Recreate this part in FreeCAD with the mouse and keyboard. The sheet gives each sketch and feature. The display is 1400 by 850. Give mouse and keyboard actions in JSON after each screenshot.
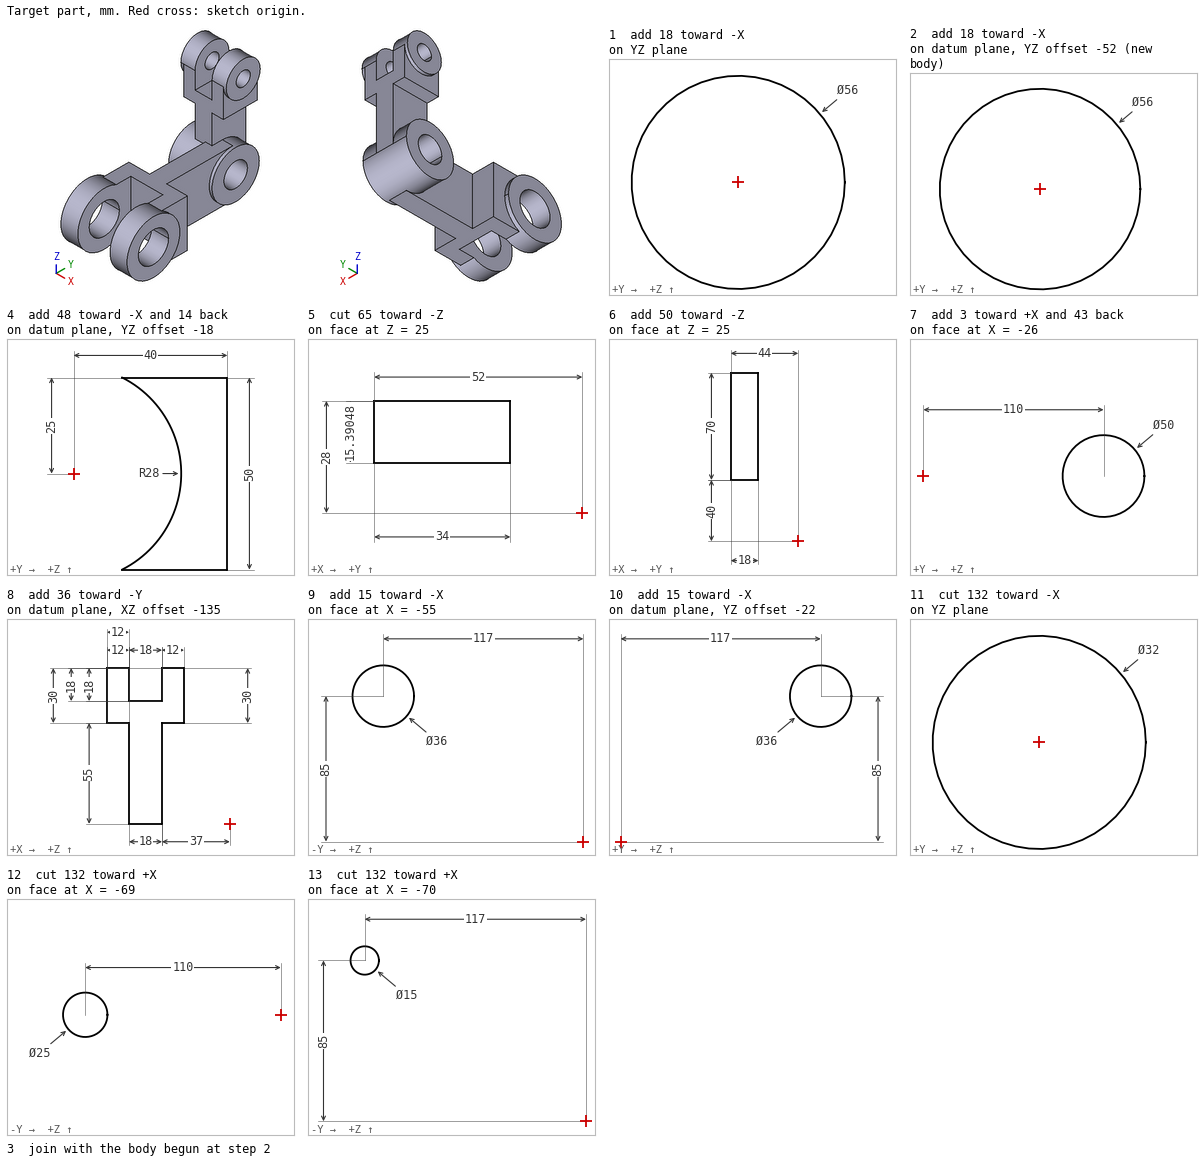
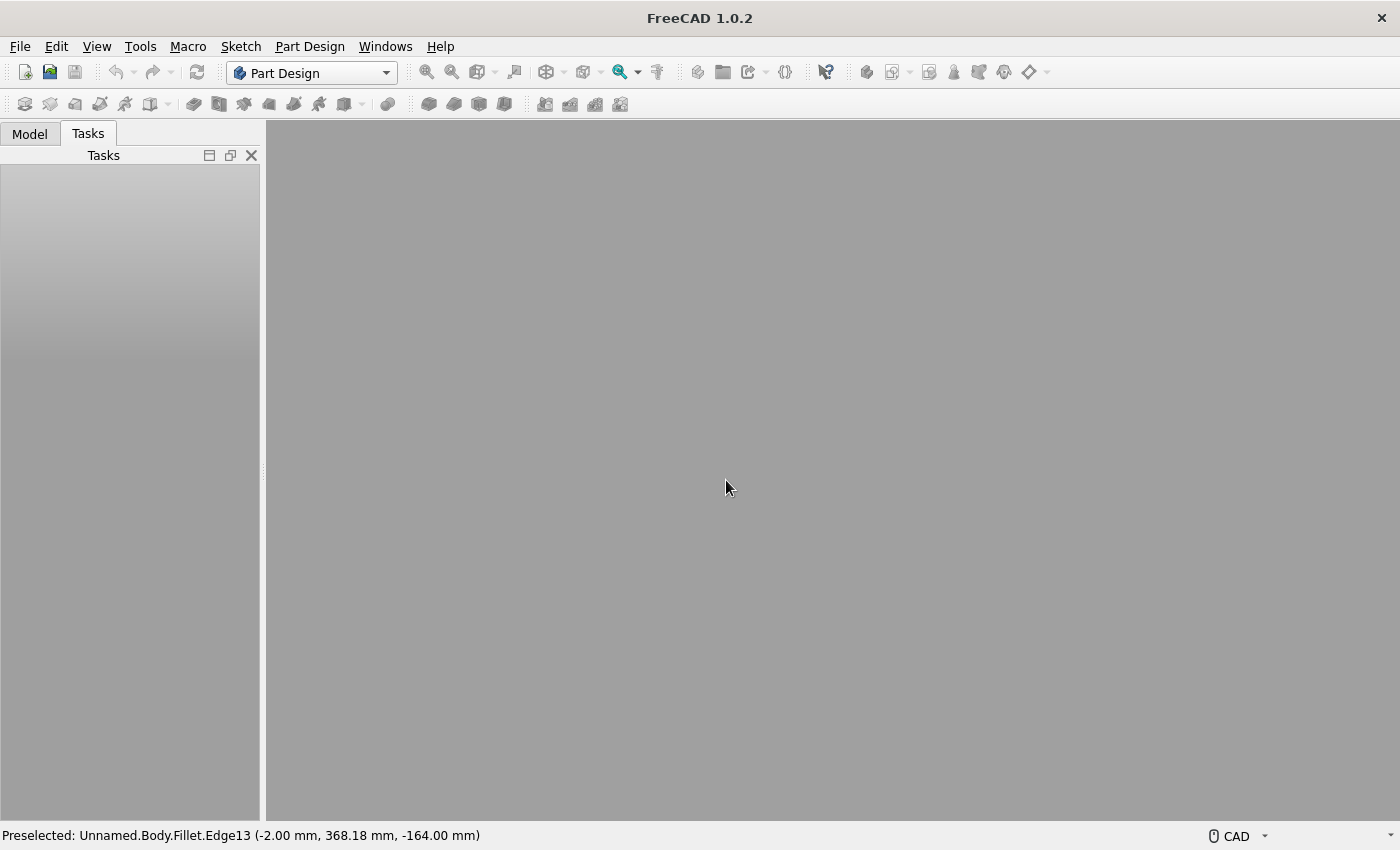
{"action": "key", "text": "ctrl+n"}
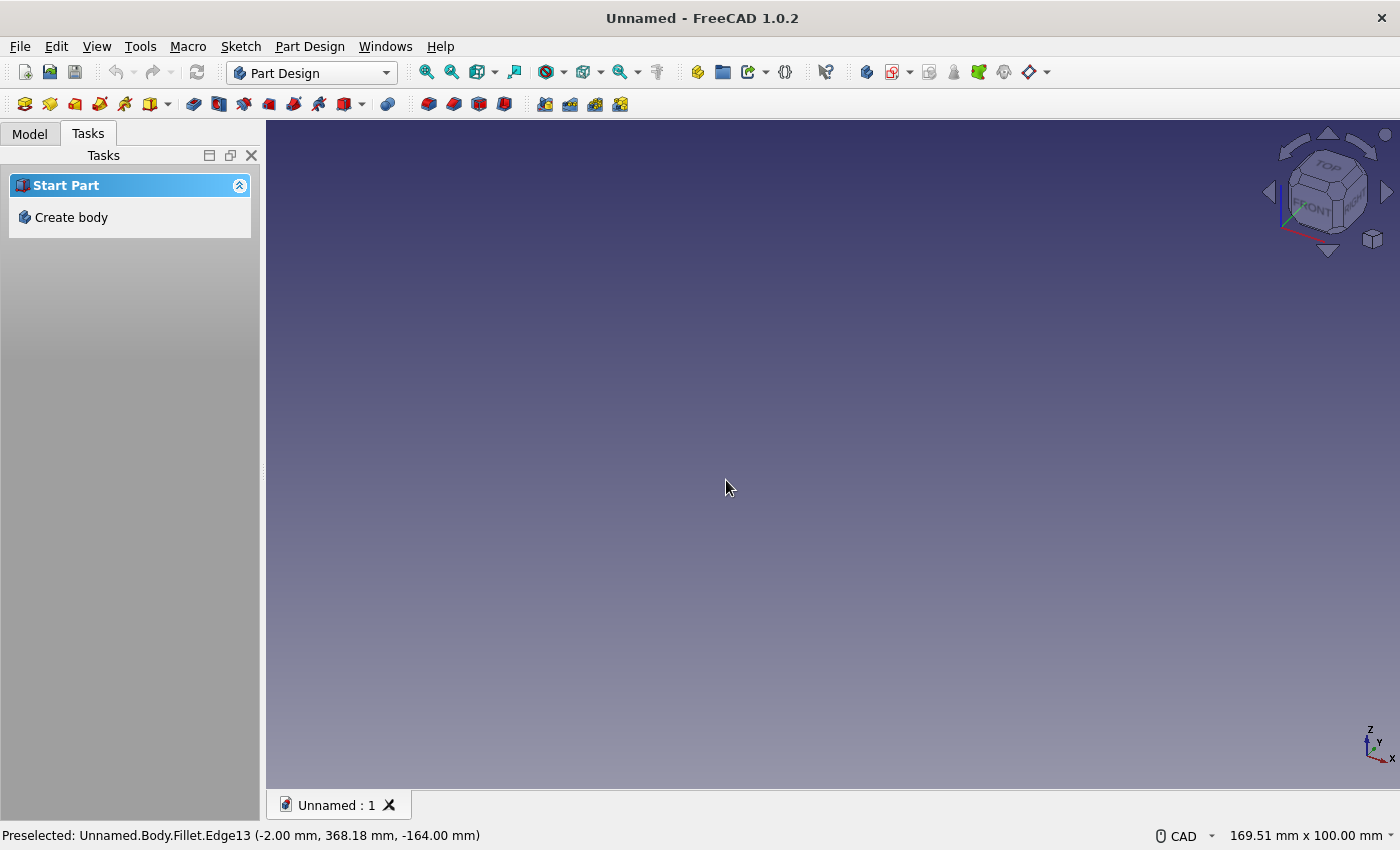
{"action": "left_click", "coordinate": [892, 72]}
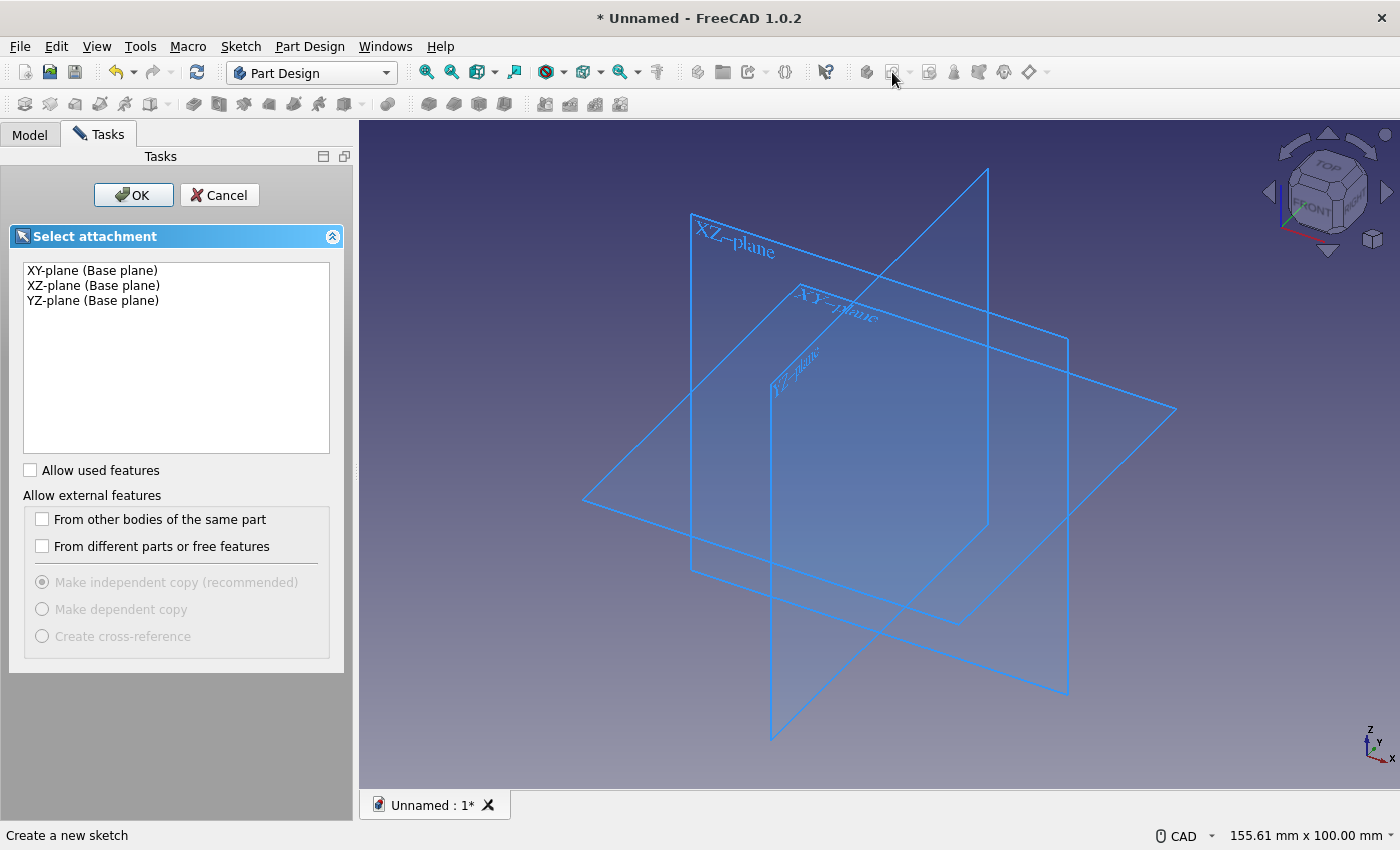
{"action": "left_click", "coordinate": [84, 300]}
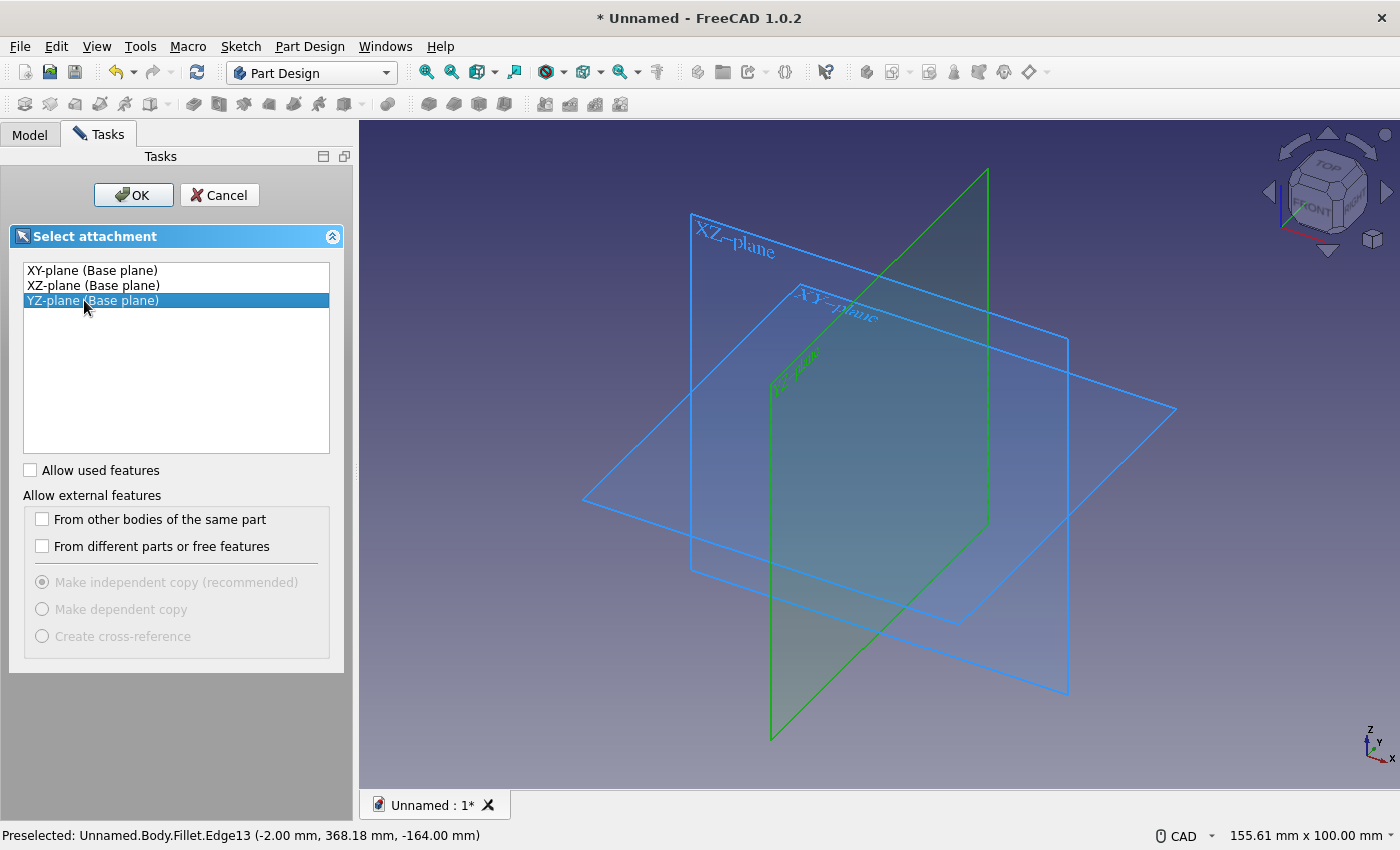
{"action": "left_click", "coordinate": [134, 195]}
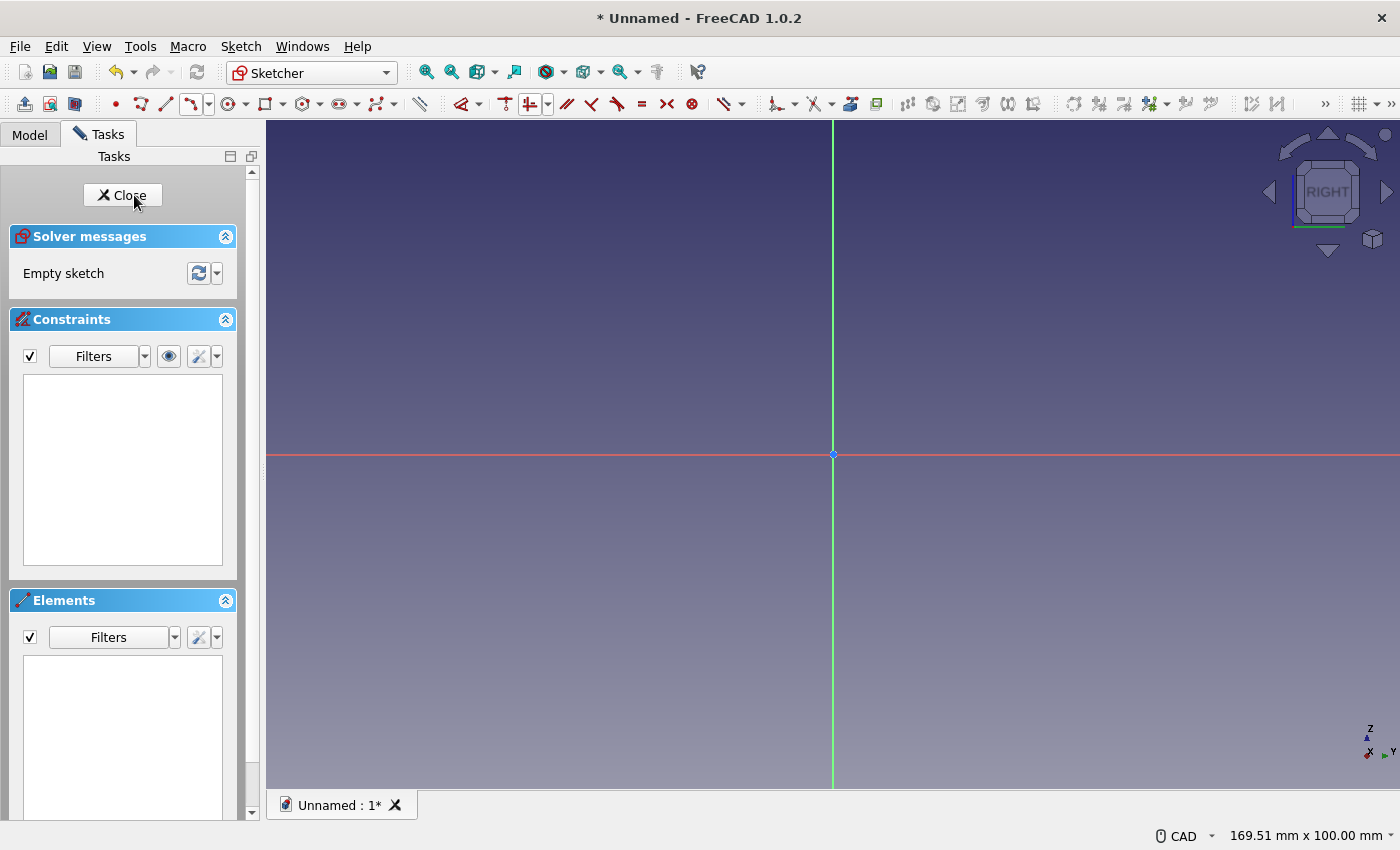
{"action": "key", "text": "g c"}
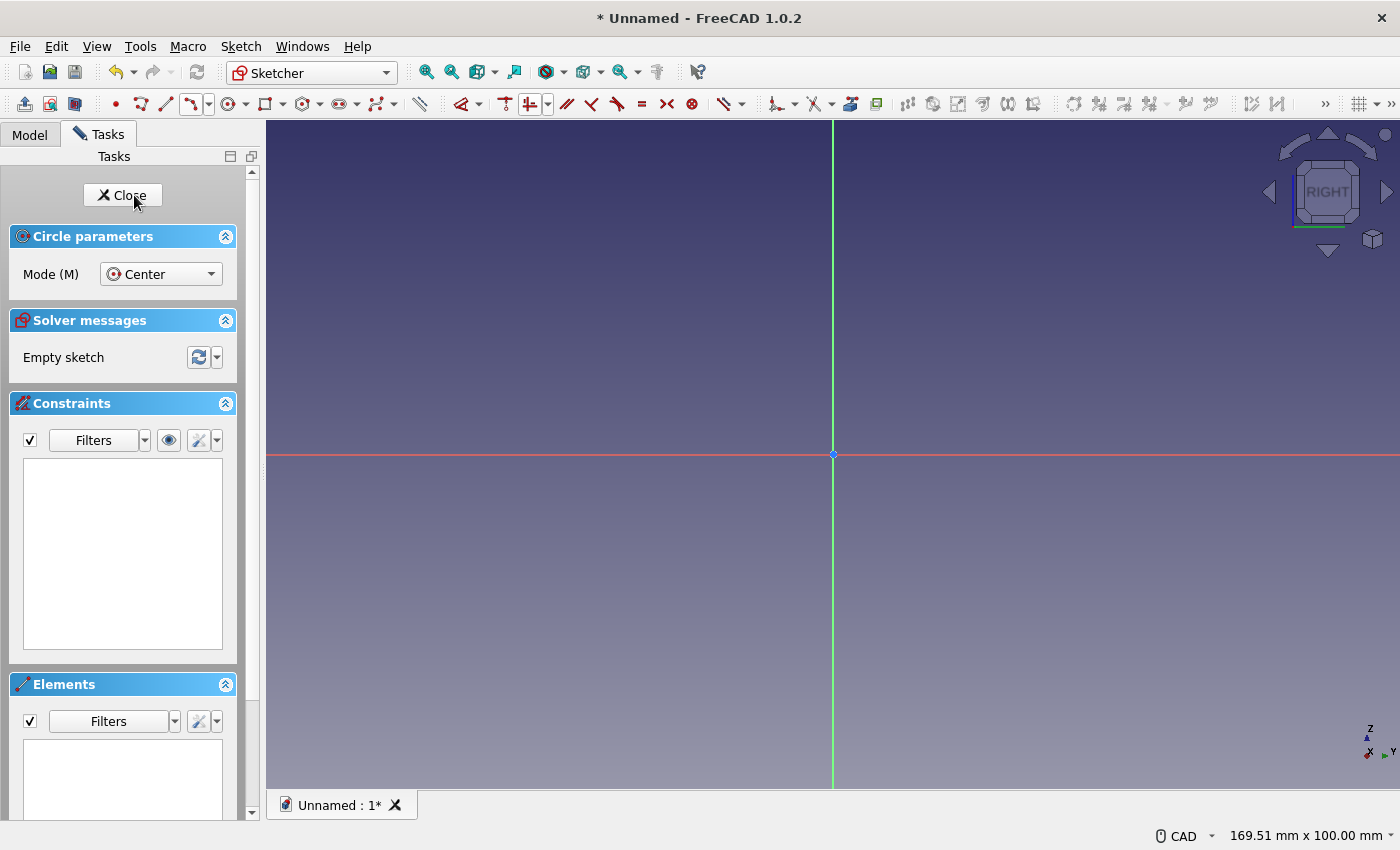
{"action": "left_click", "coordinate": [833, 454]}
{"action": "left_click", "coordinate": [965, 322]}
{"action": "key", "text": "Escape"}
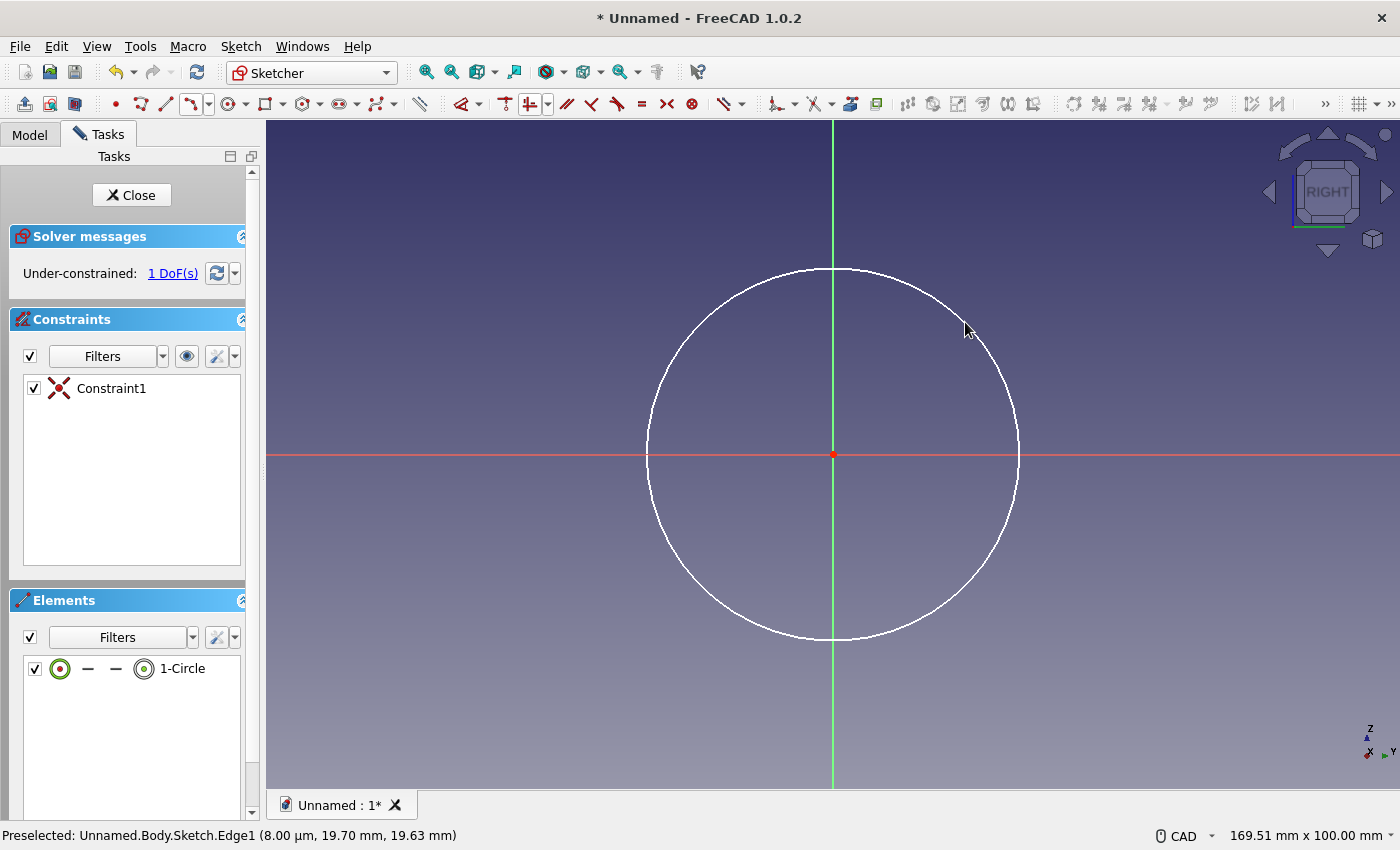
{"action": "left_click", "coordinate": [964, 322]}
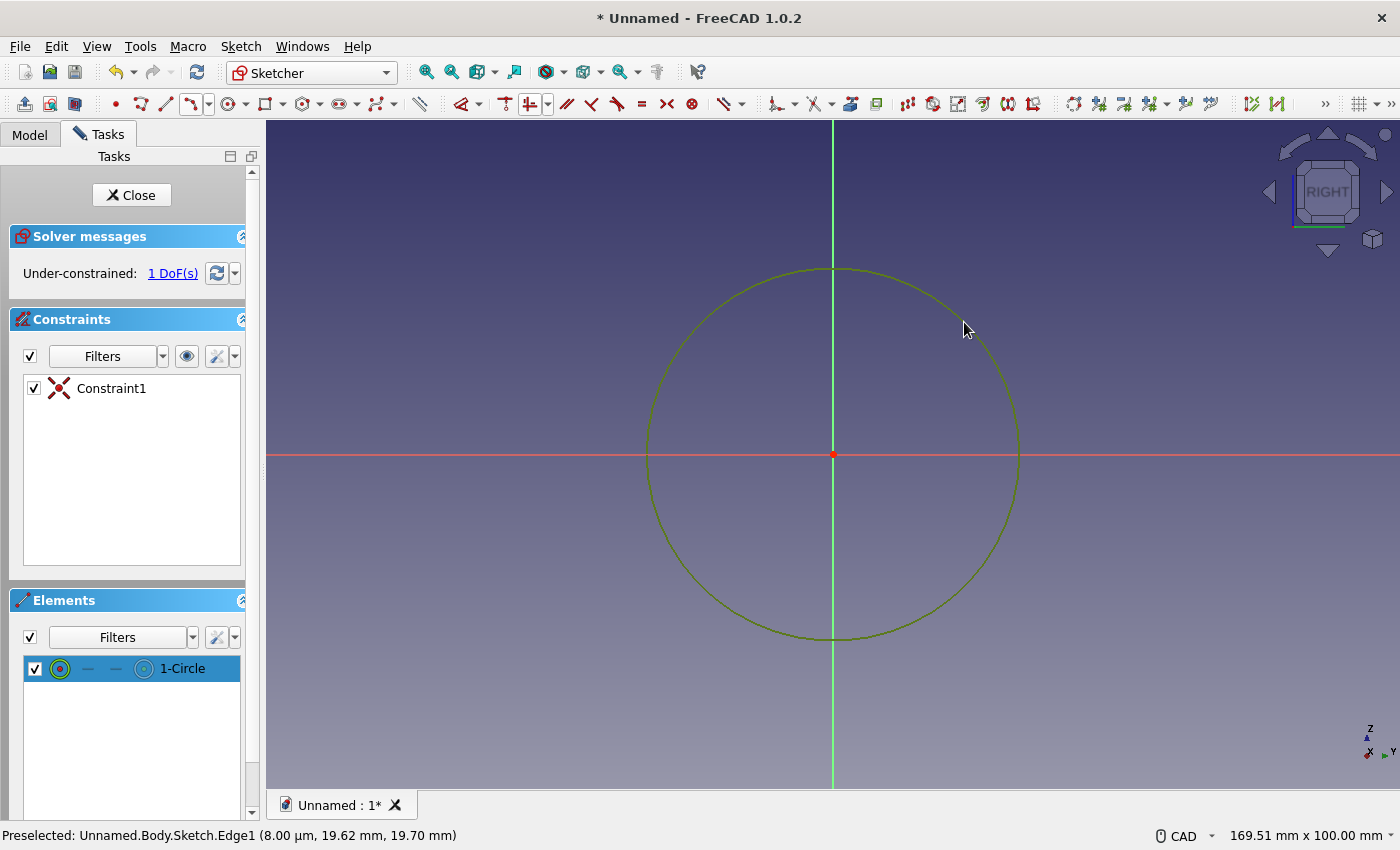
{"action": "key", "text": "k o"}